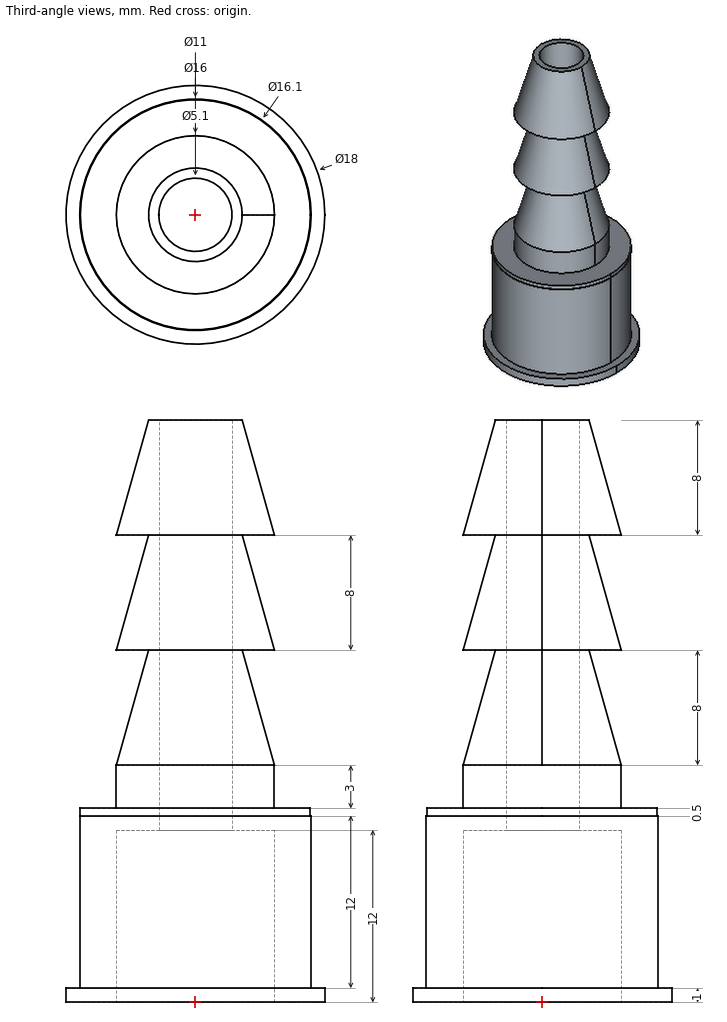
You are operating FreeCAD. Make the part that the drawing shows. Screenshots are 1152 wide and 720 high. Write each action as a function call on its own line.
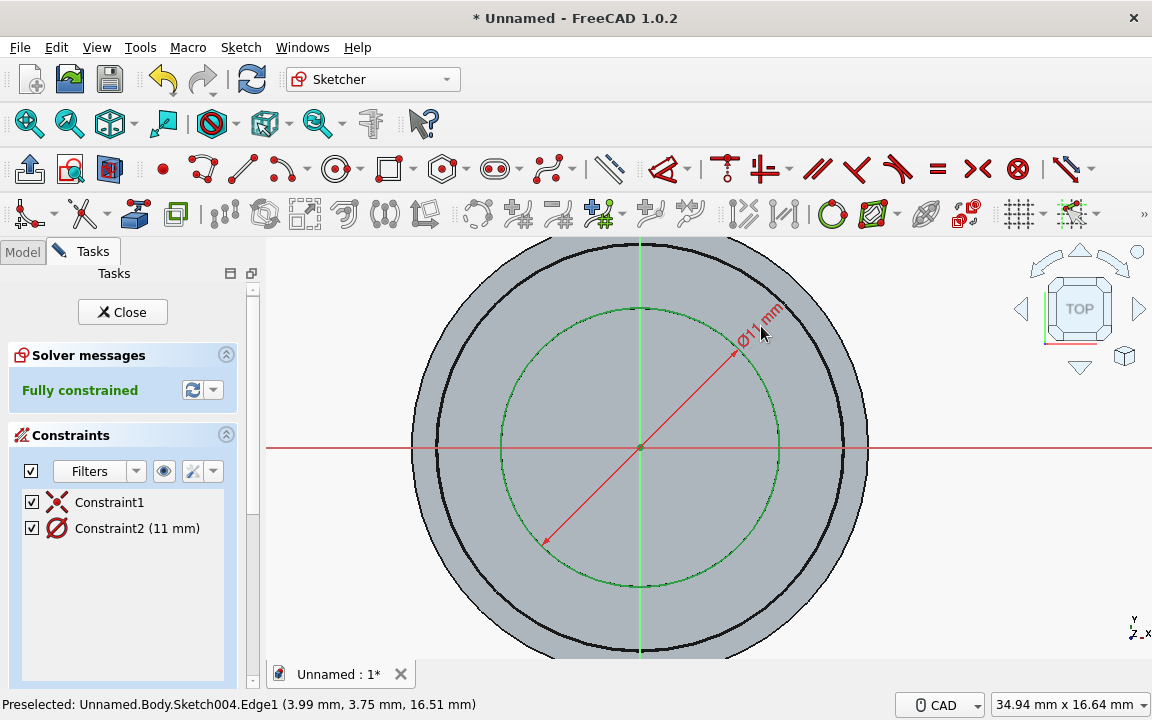
click(123, 312)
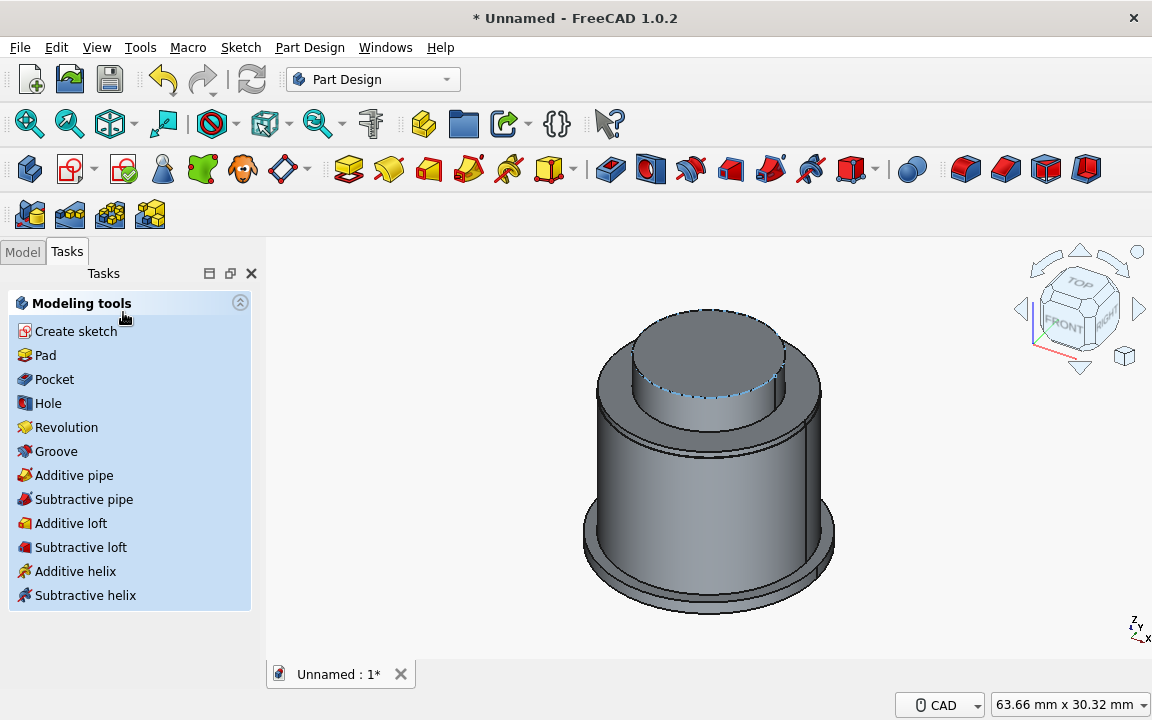
click(350, 170)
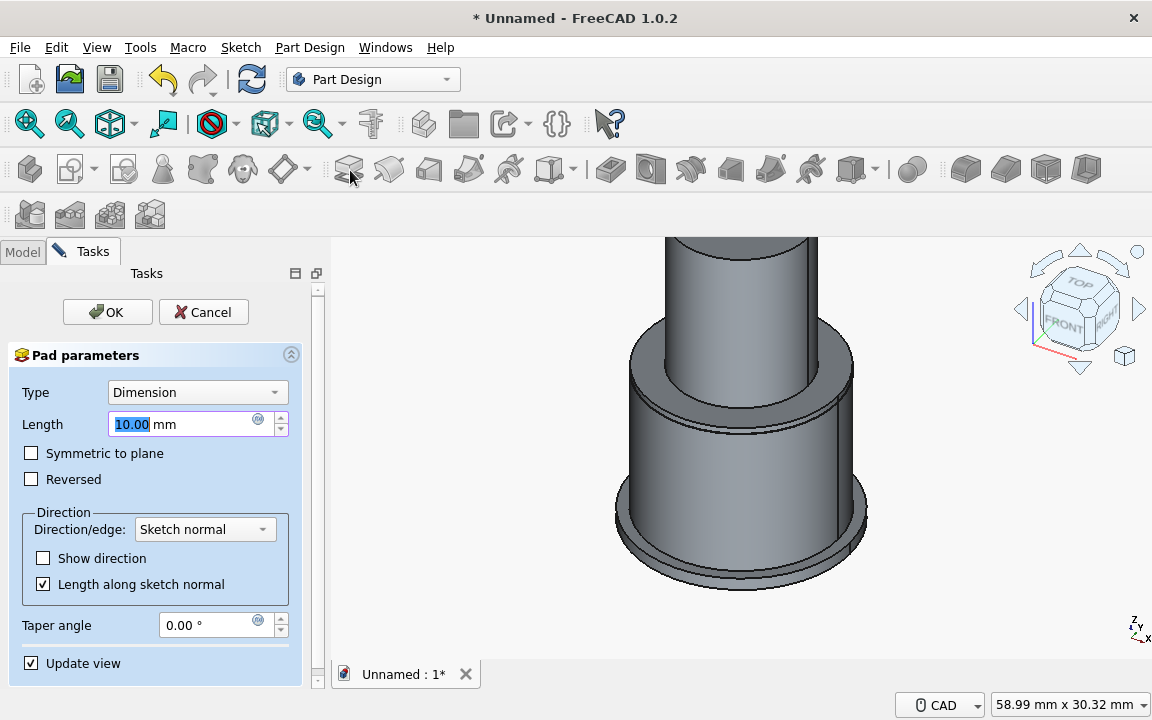
text(8)
key(Tab)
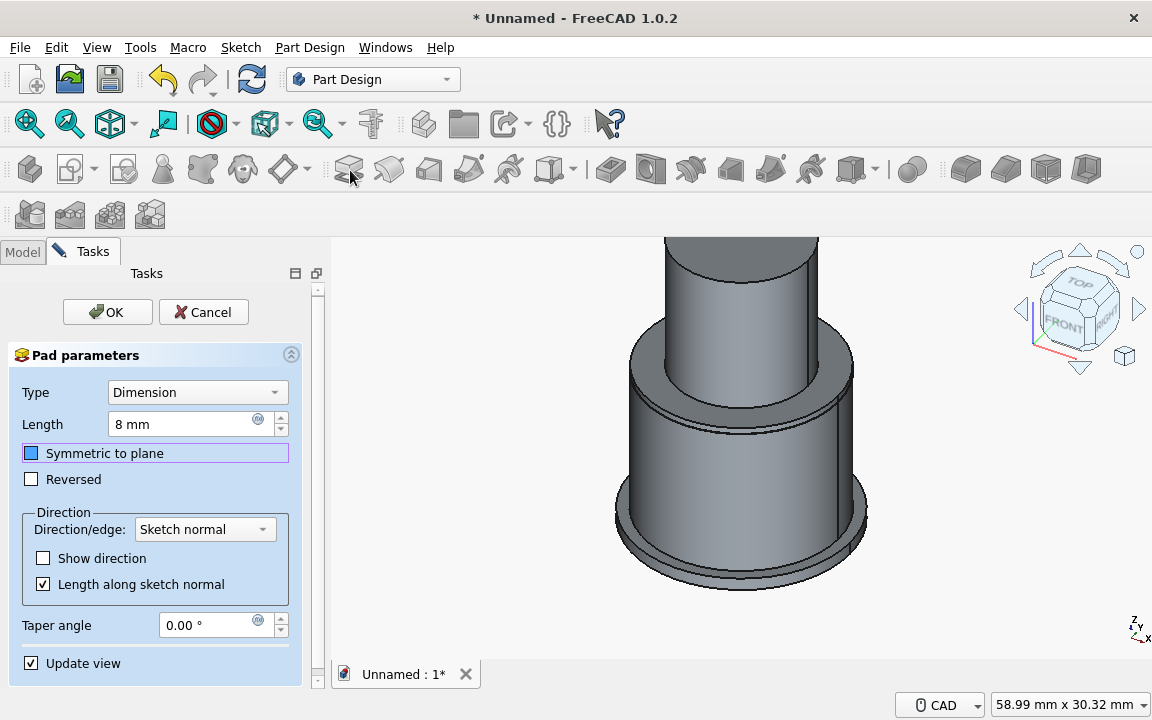
triple_click(216, 625)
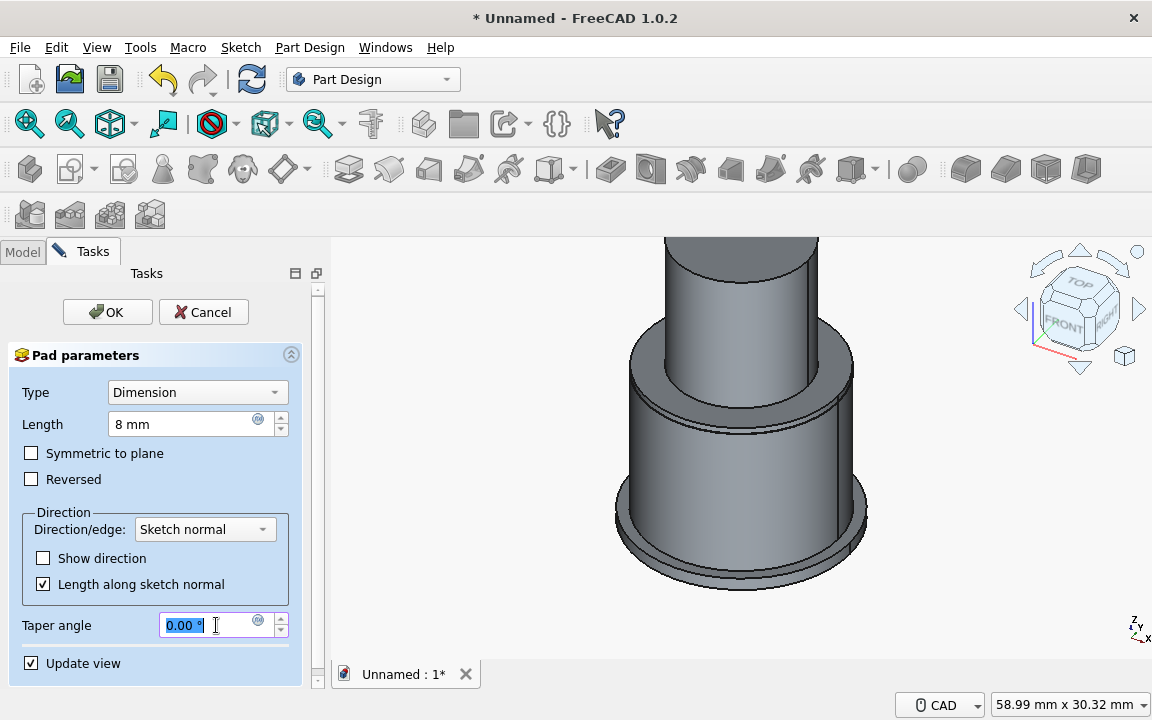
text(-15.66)
key(Tab)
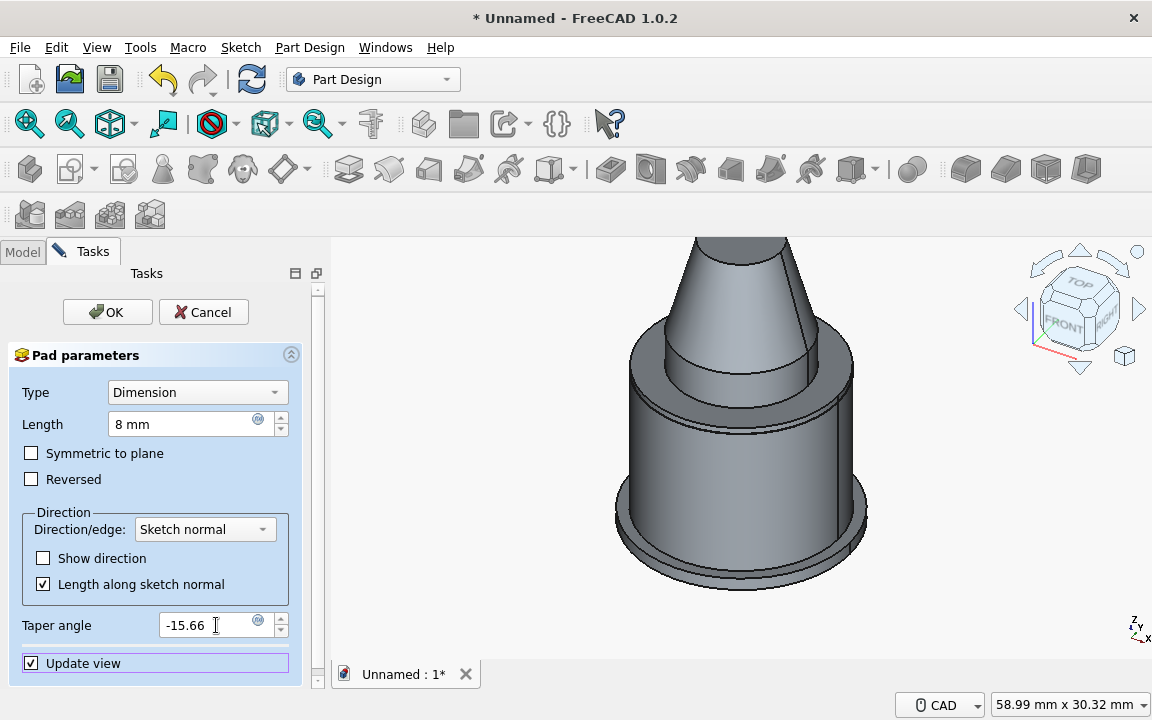
click(108, 312)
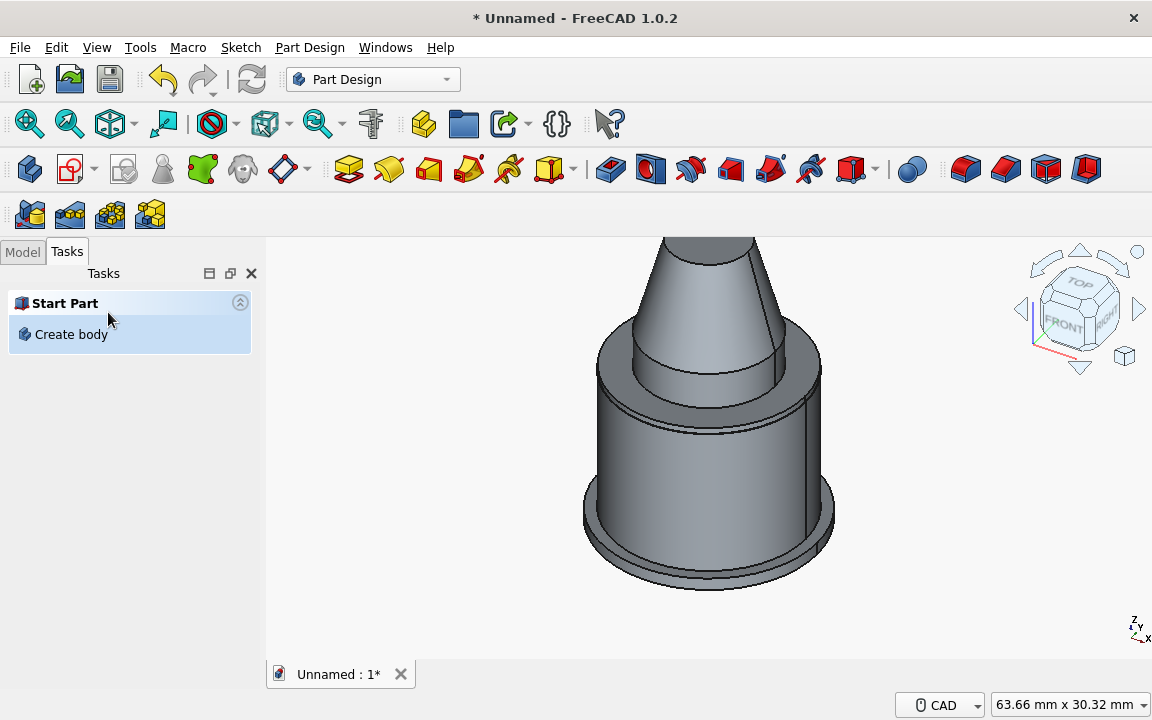
key(v)
key(f)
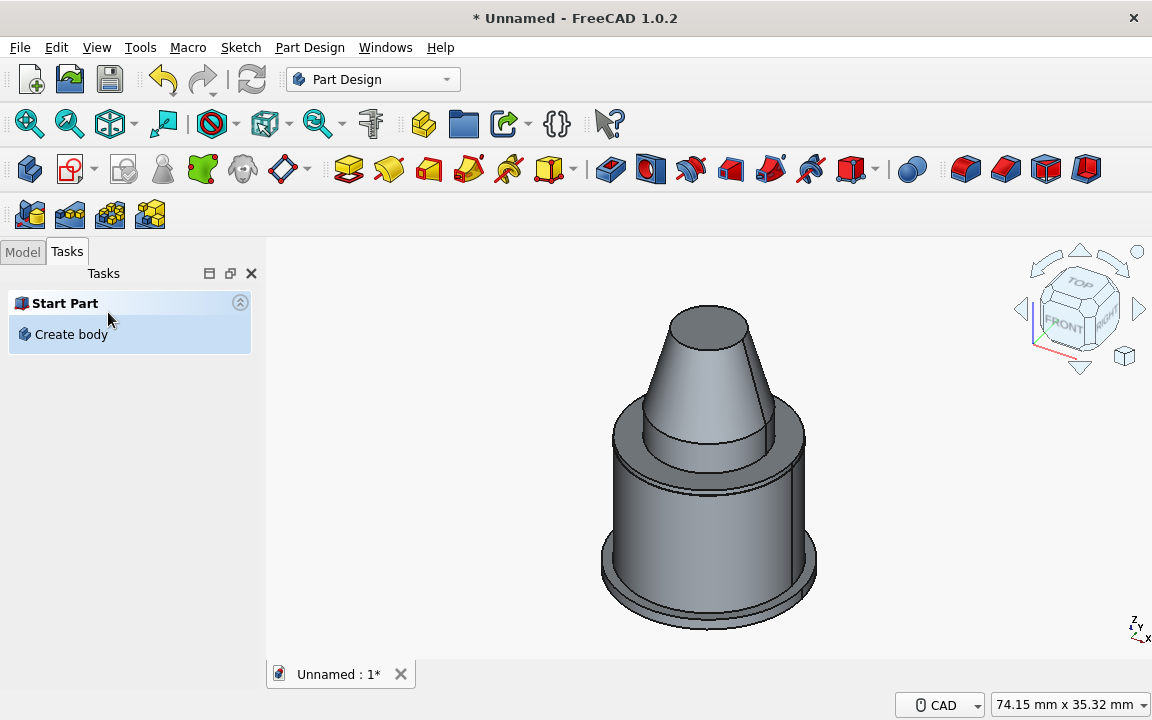
click(709, 327)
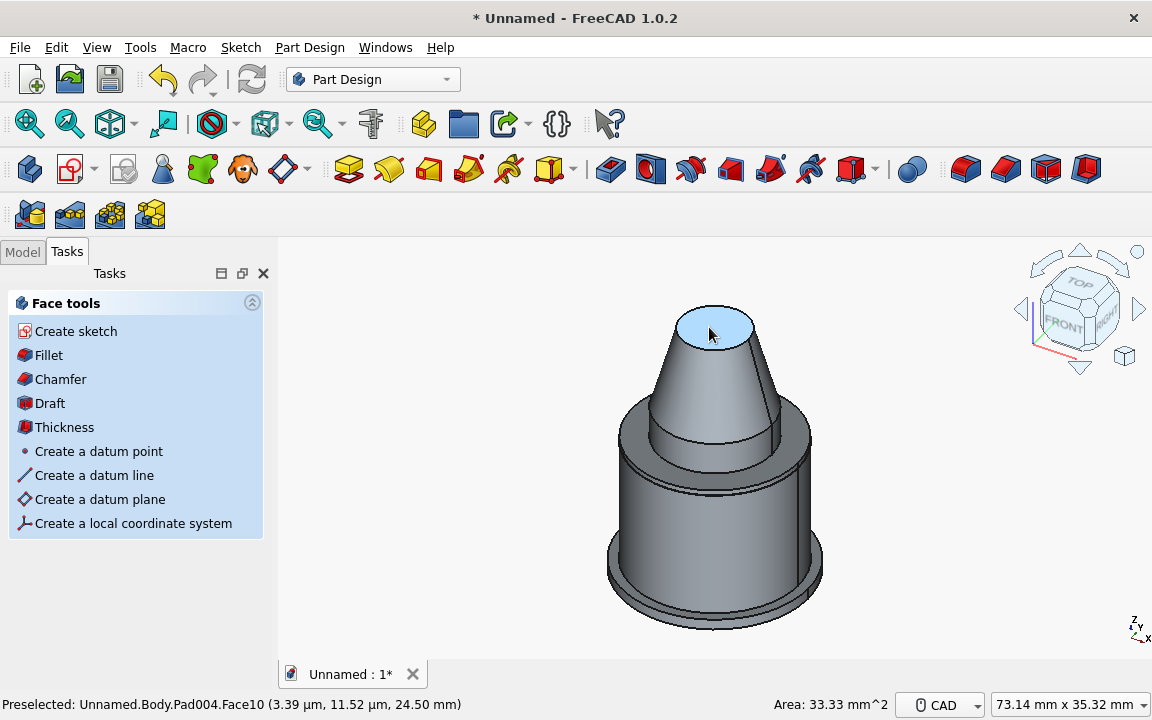
click(70, 170)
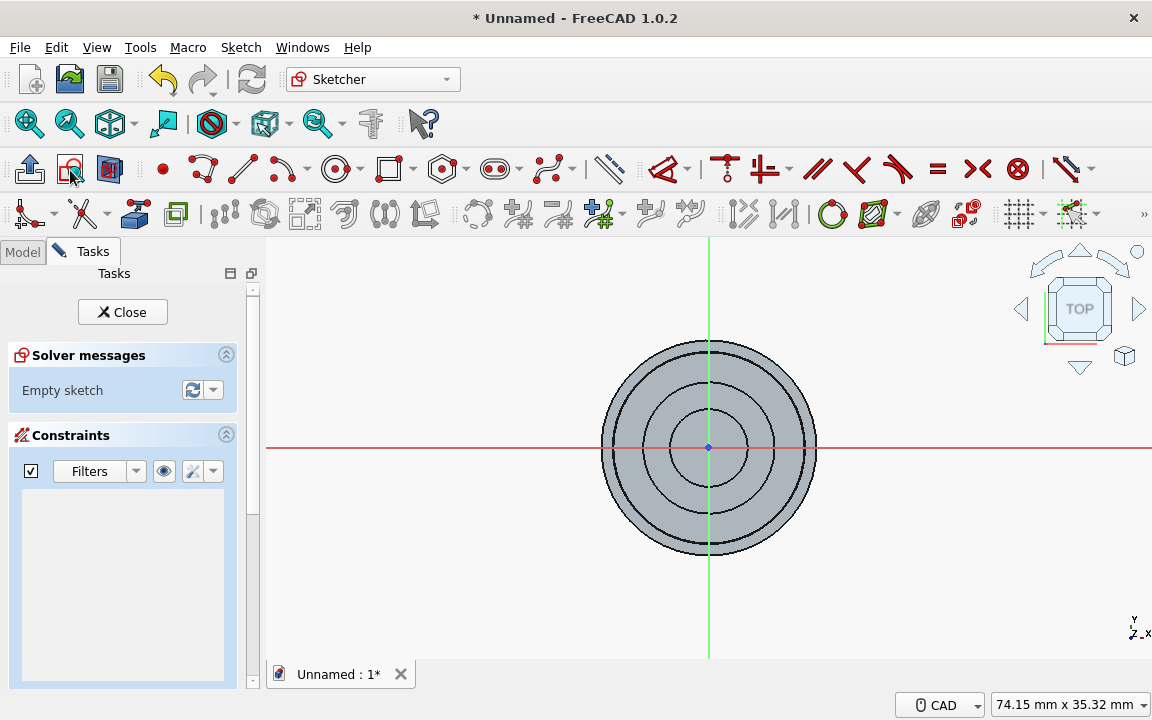
scroll(792, 448, up, 3)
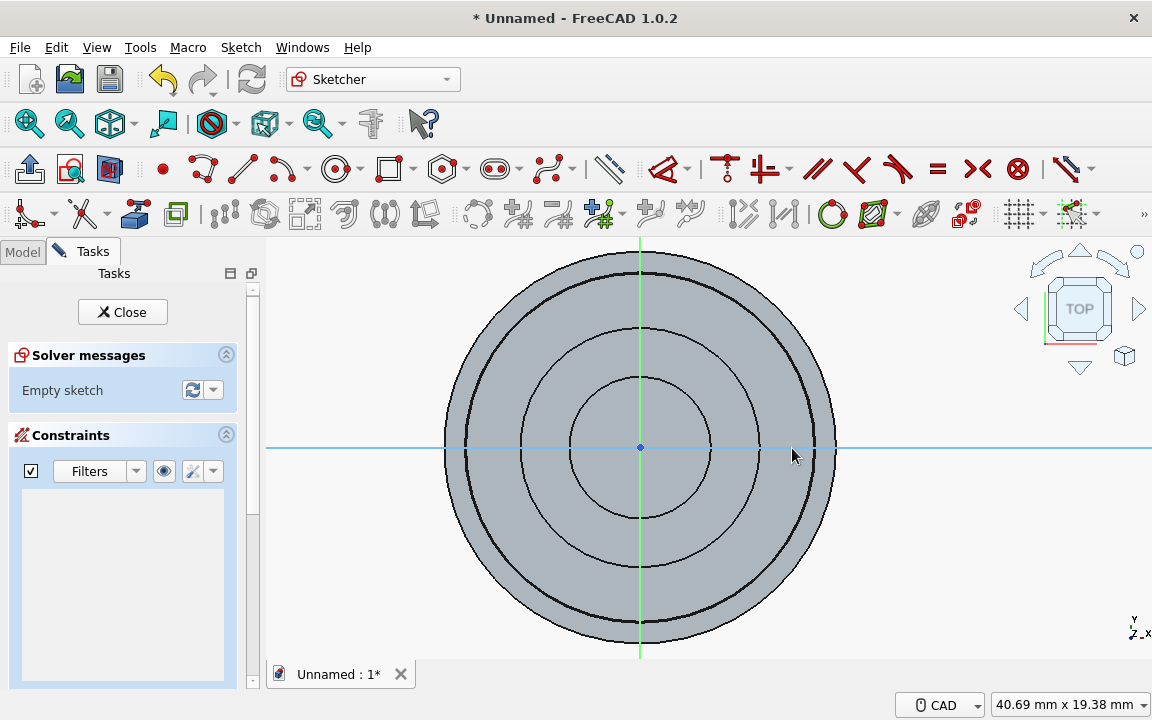
click(336, 170)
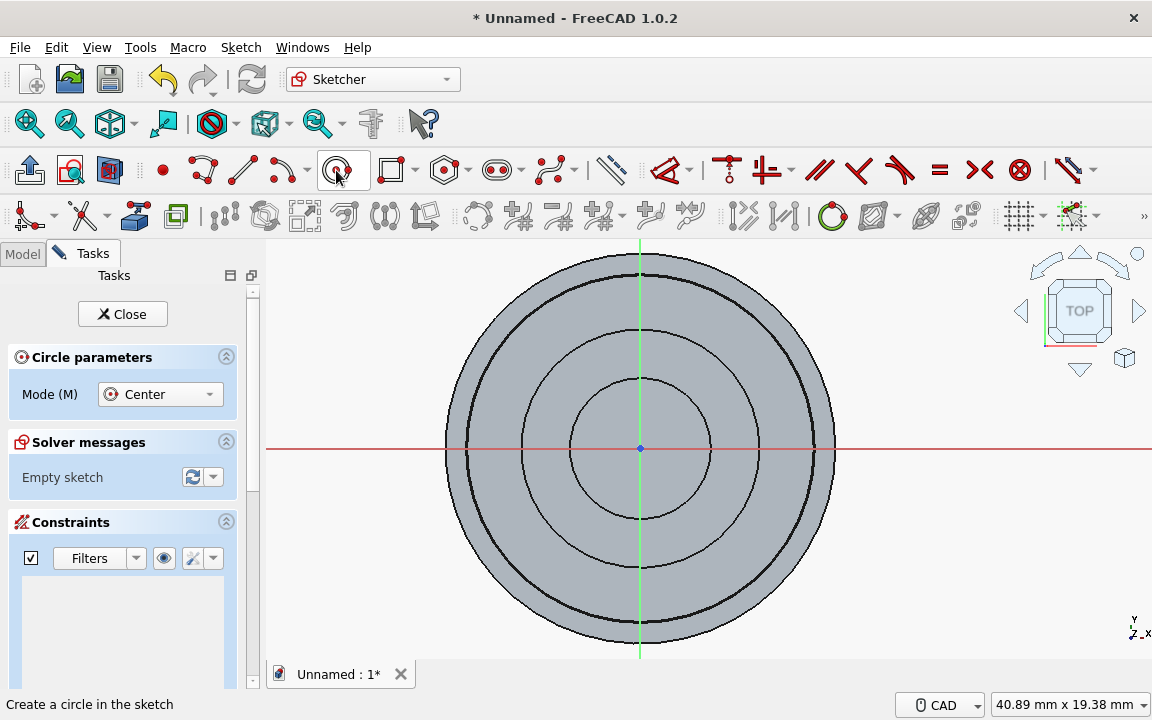
click(640, 449)
click(725, 364)
key(Escape)